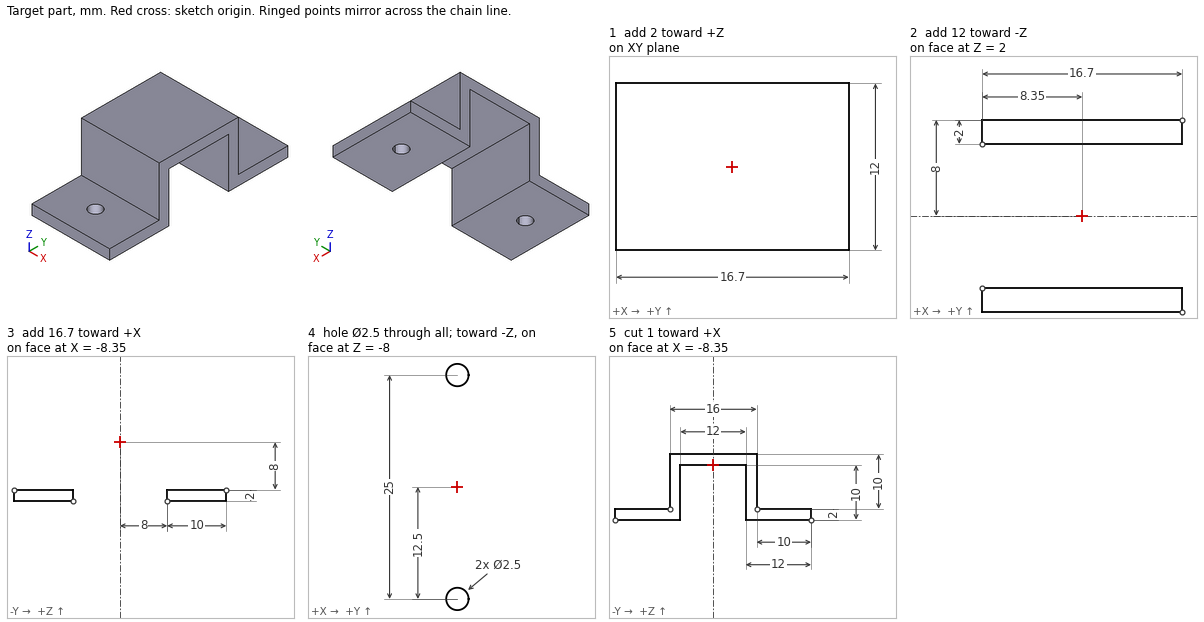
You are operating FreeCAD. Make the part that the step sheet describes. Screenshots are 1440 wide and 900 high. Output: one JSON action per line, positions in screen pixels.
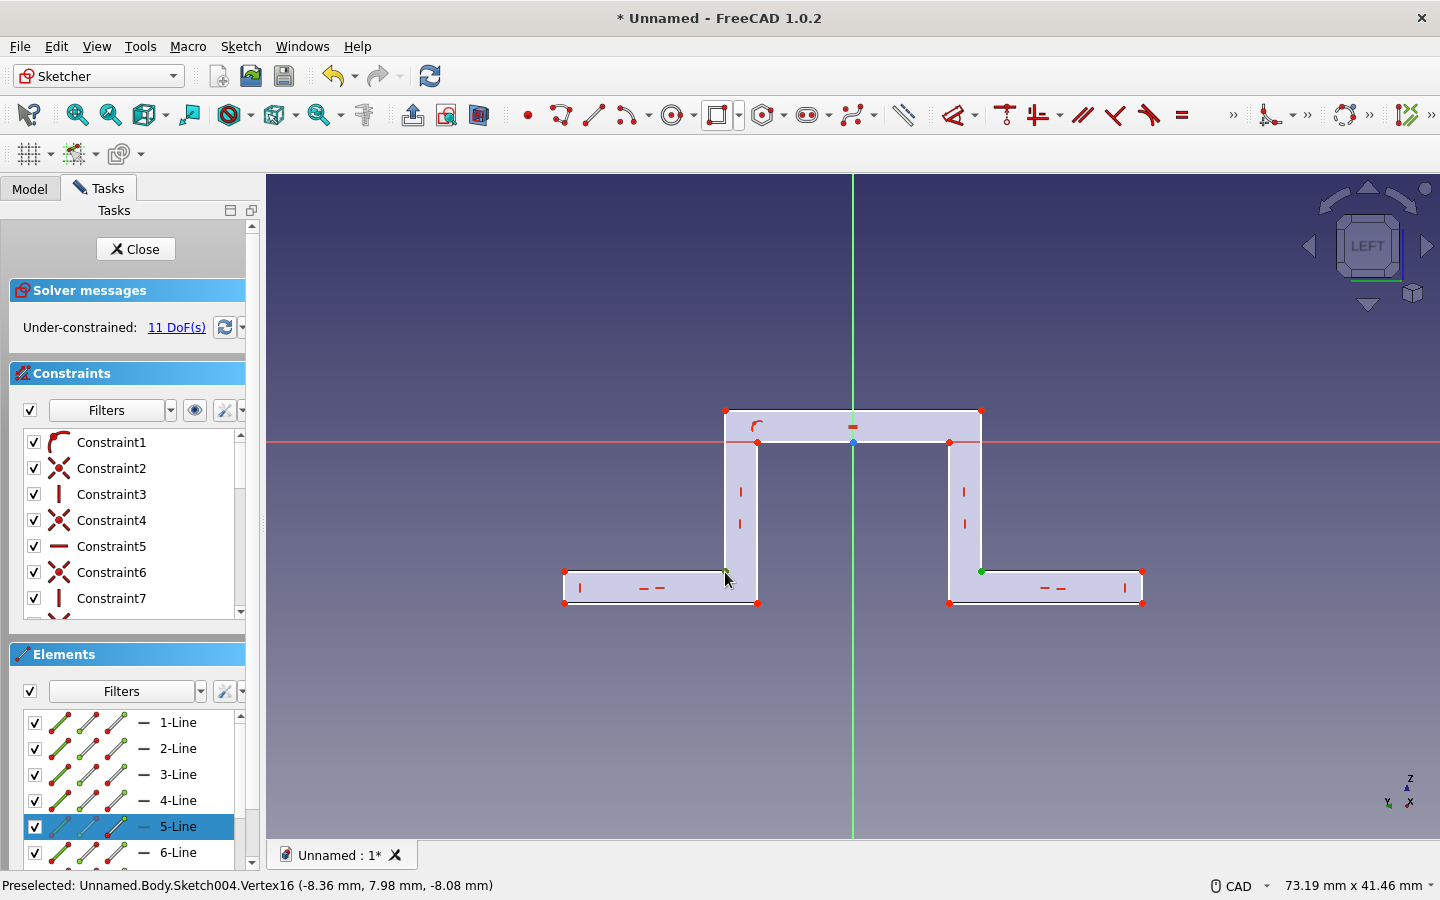
{"action": "left_click", "coordinate": [853, 768]}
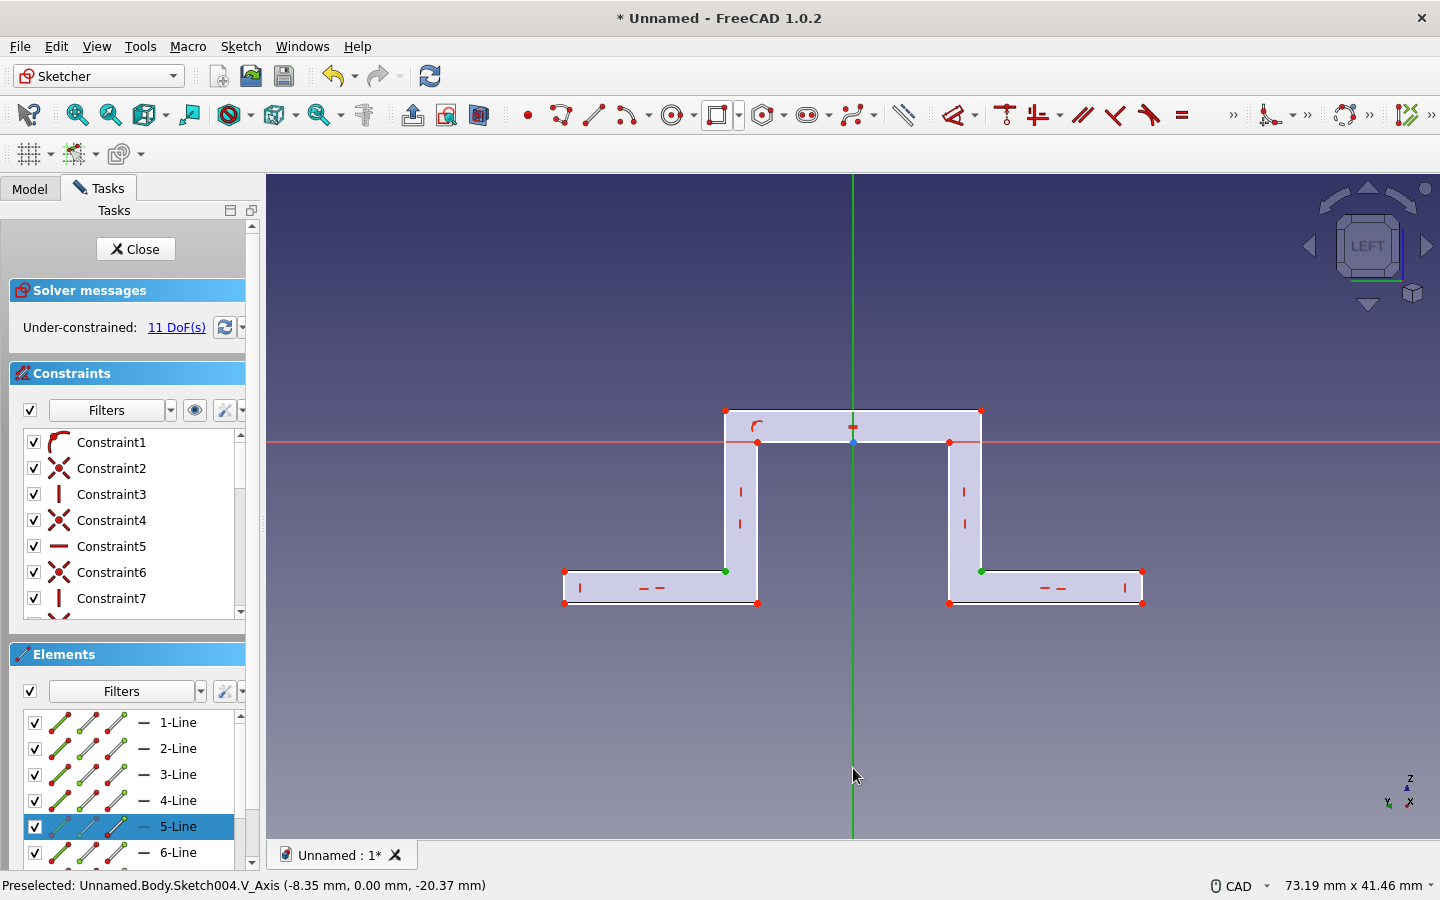
{"action": "key", "text": "s"}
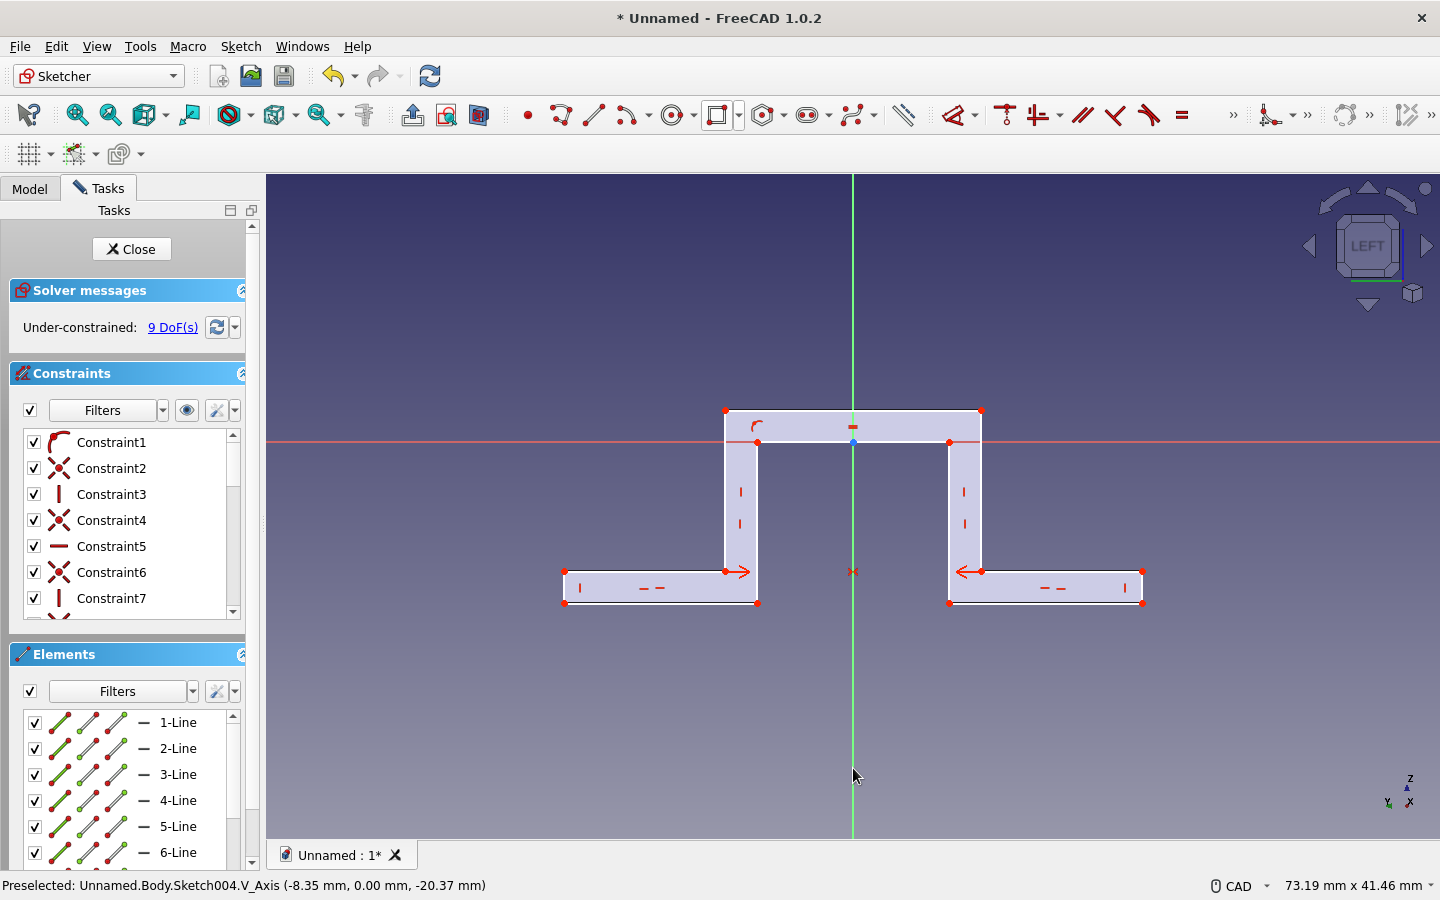
{"action": "left_click", "coordinate": [1142, 604]}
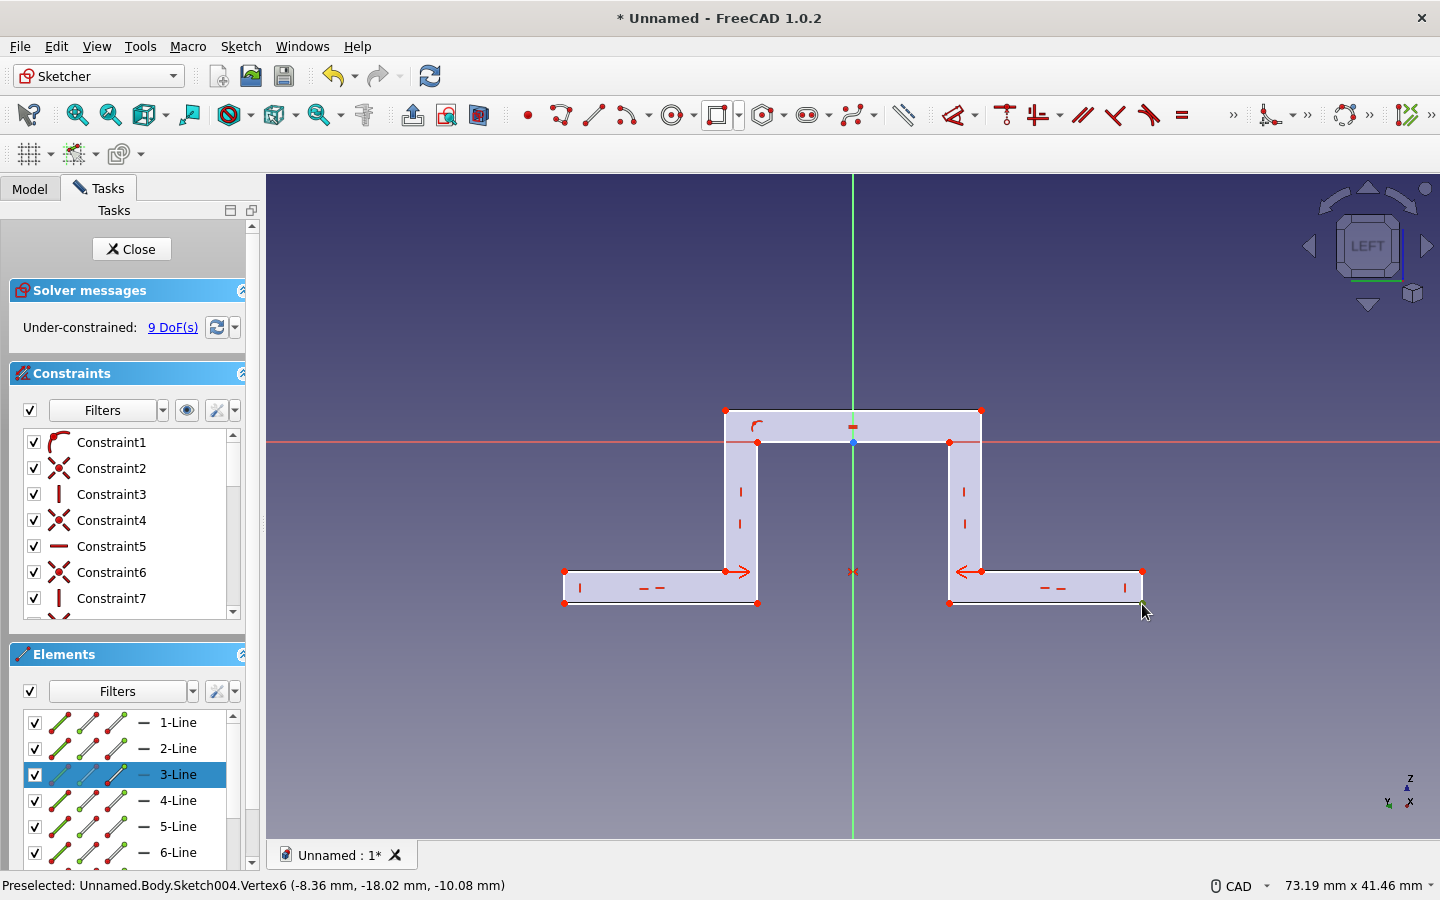
{"action": "left_click", "coordinate": [564, 604]}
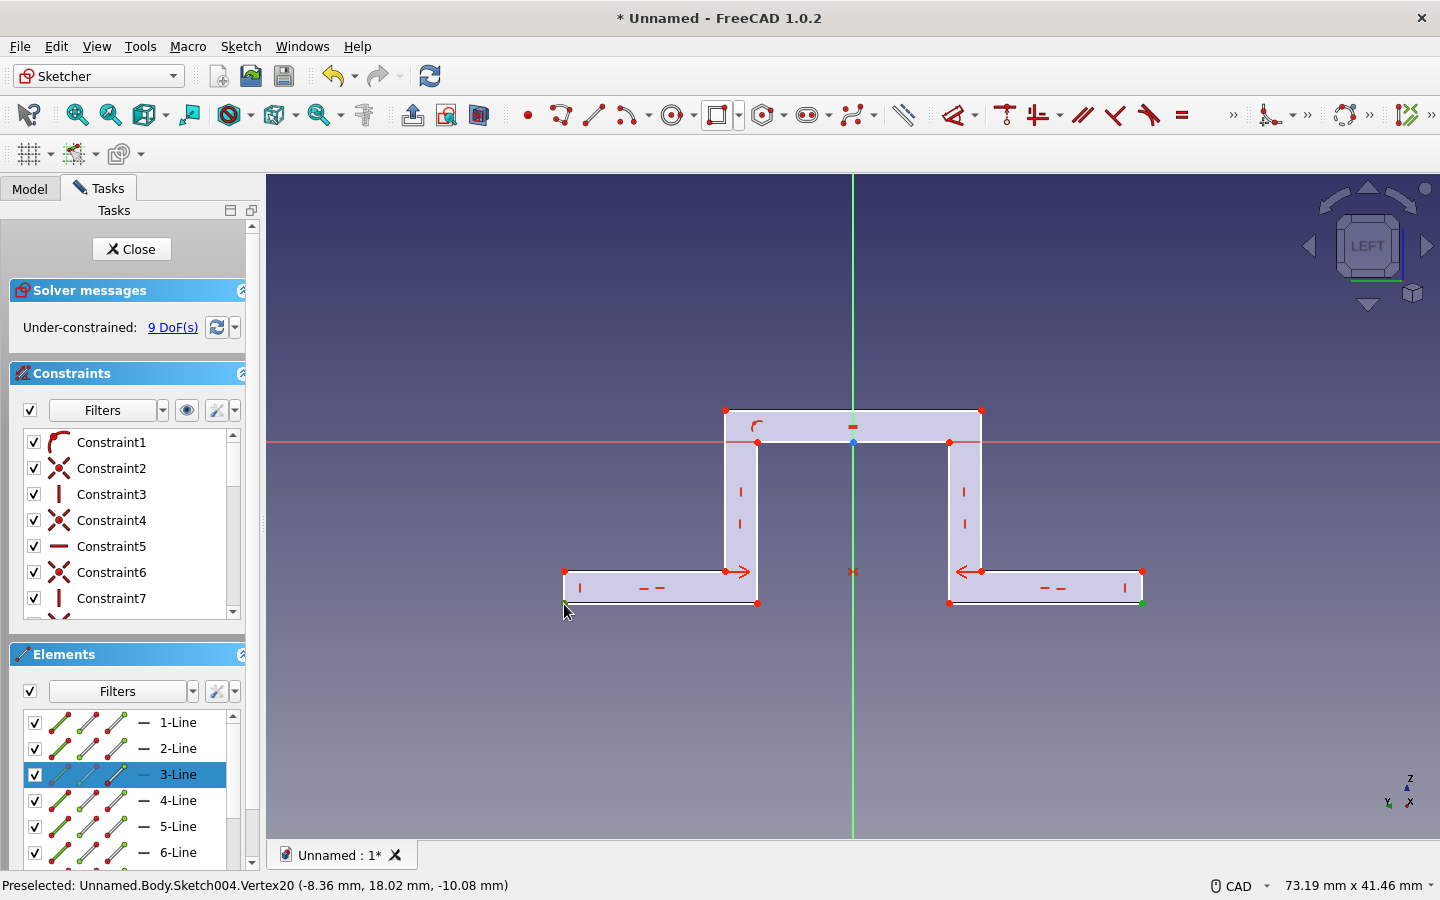
{"action": "left_click", "coordinate": [853, 768]}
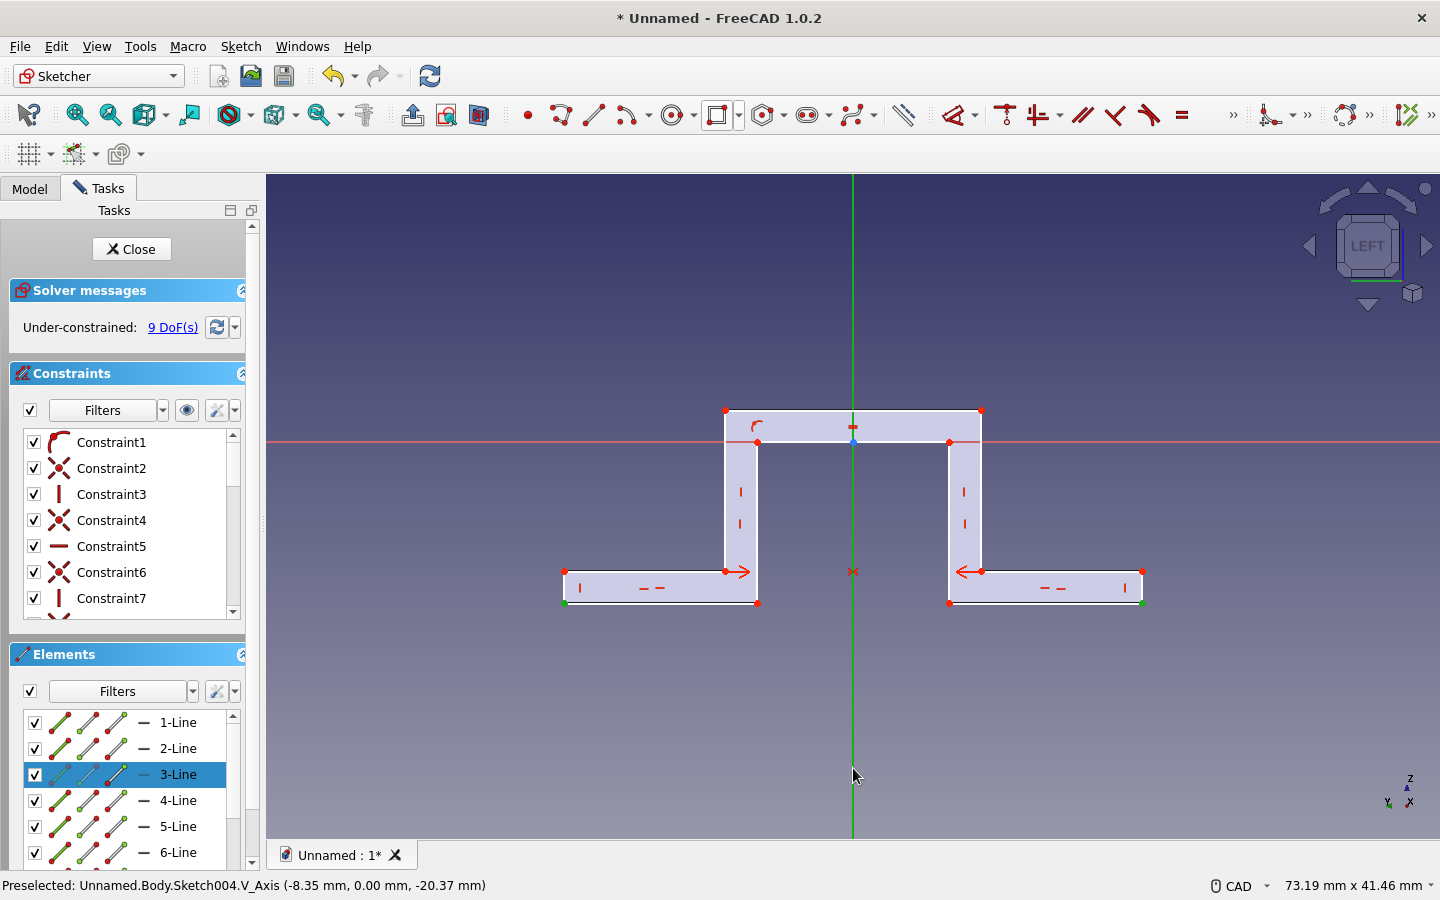
{"action": "key", "text": "s"}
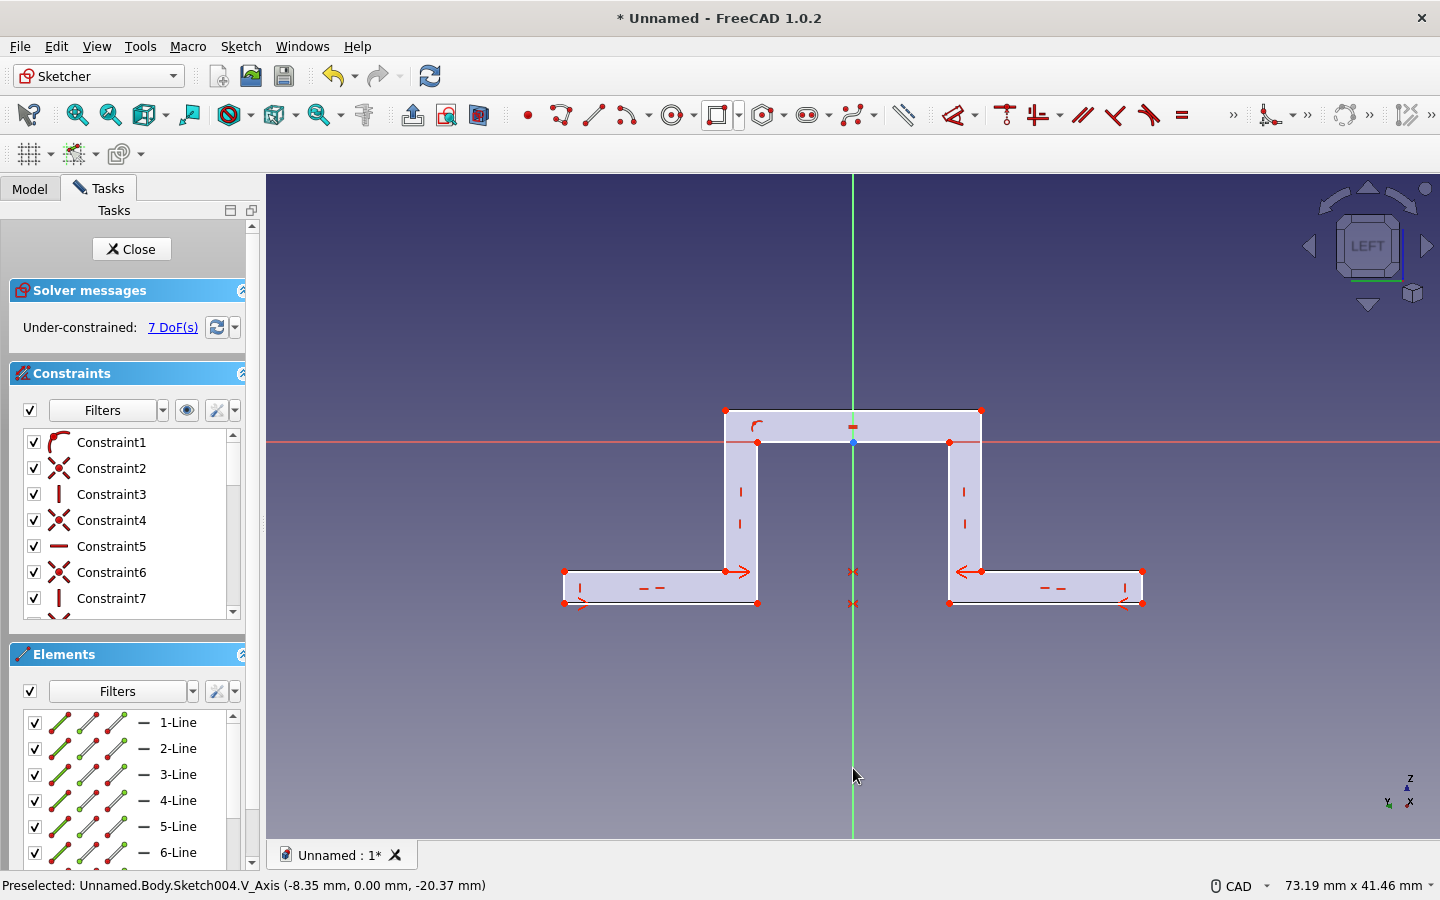
{"action": "left_click", "coordinate": [952, 116]}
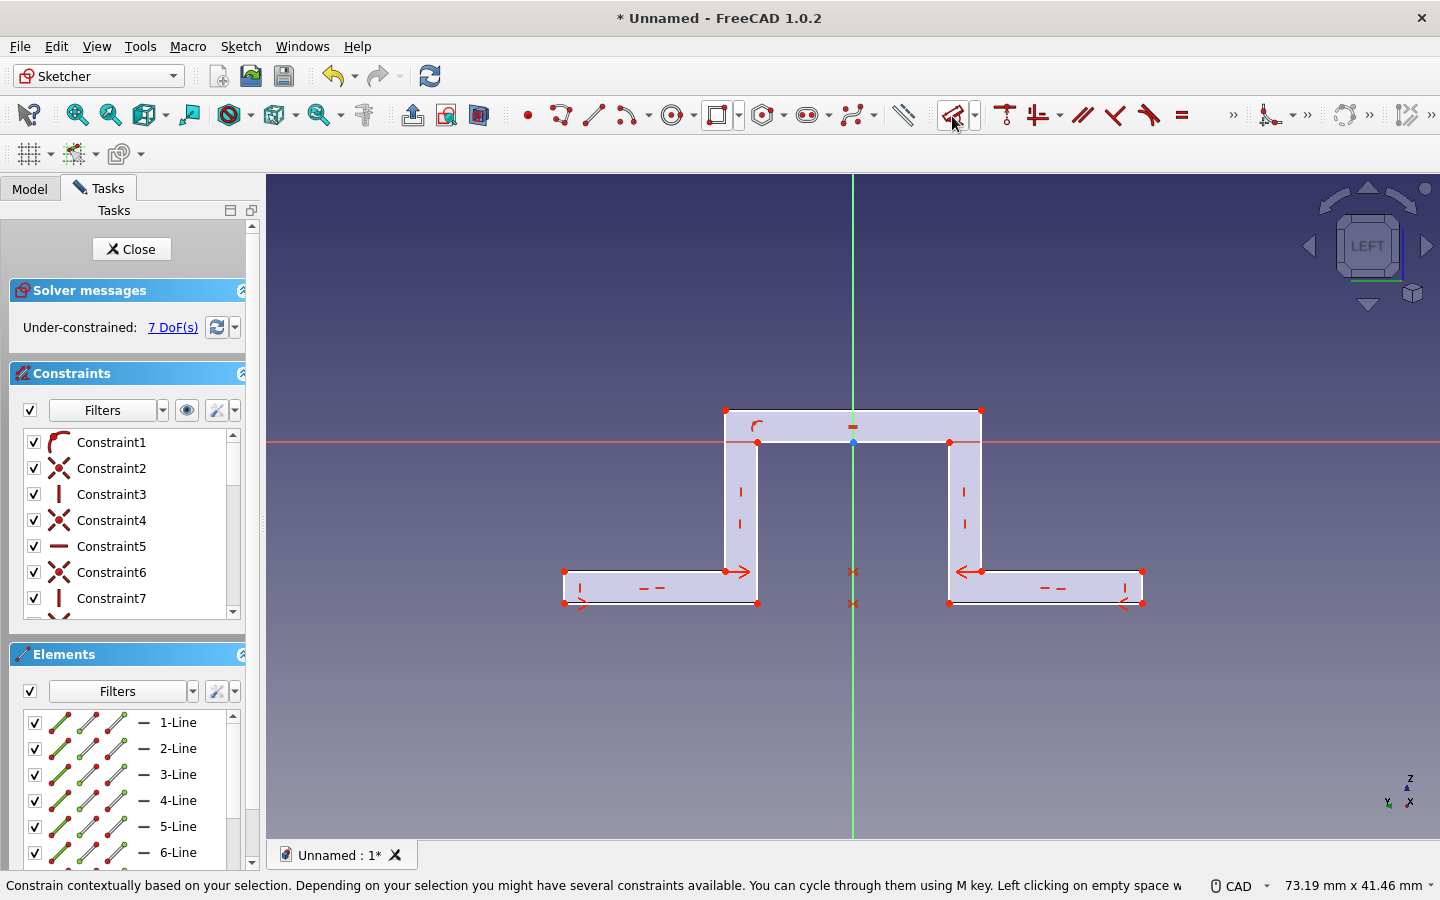
{"action": "scroll", "coordinate": [1142, 594], "scroll_direction": "up", "scroll_amount": 2}